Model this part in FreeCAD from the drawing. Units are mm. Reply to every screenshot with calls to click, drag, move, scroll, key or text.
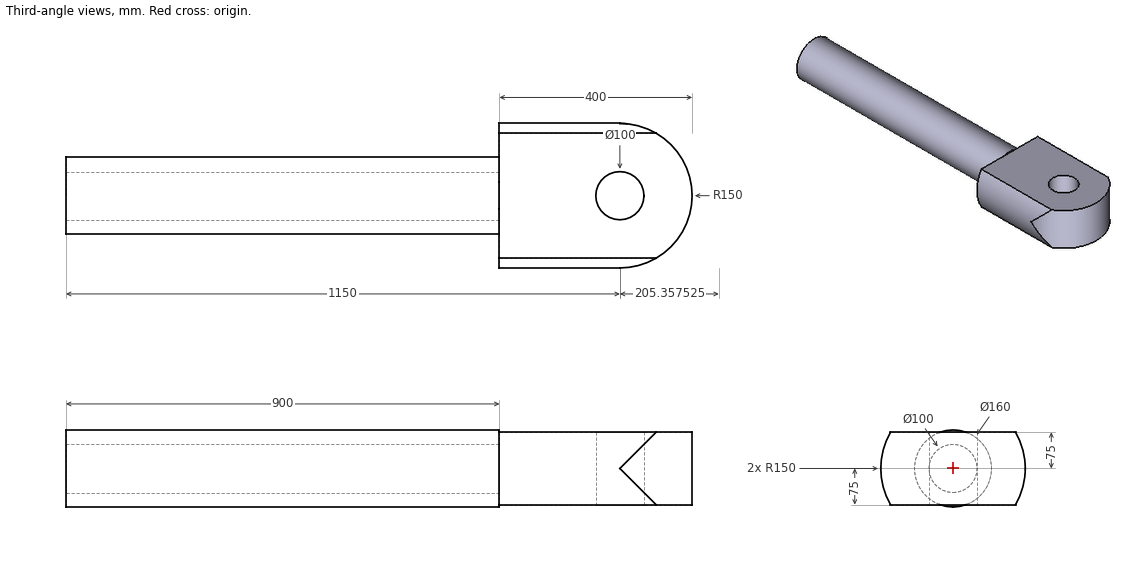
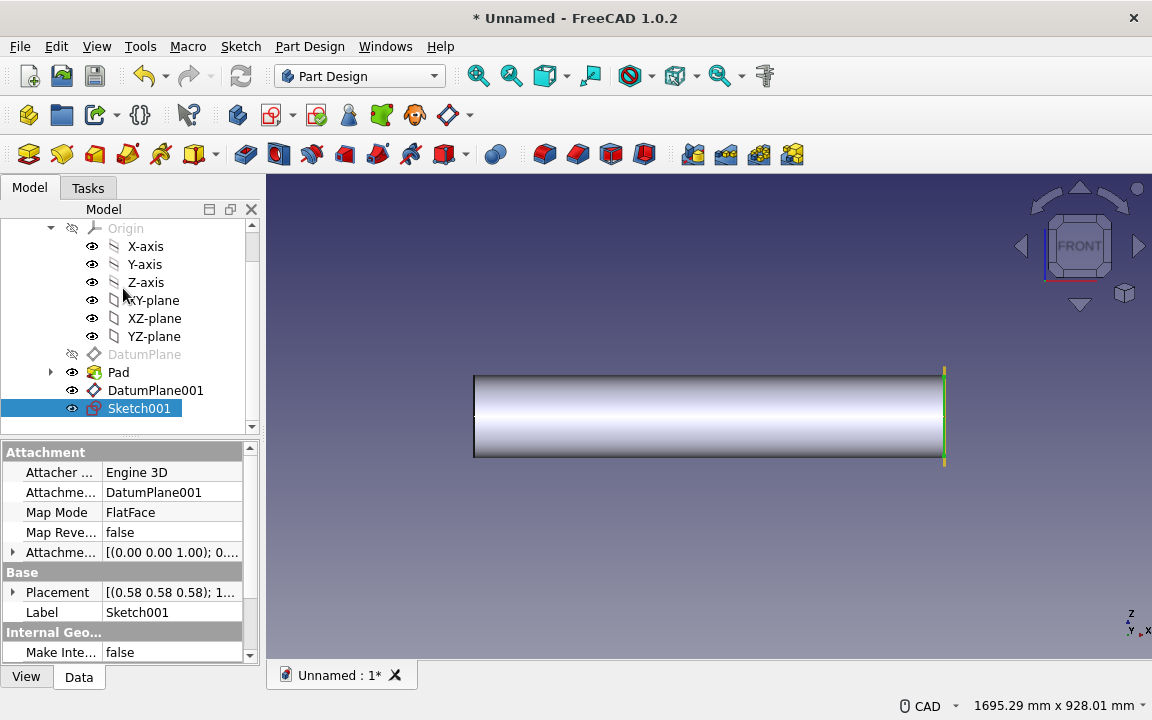
click(29, 154)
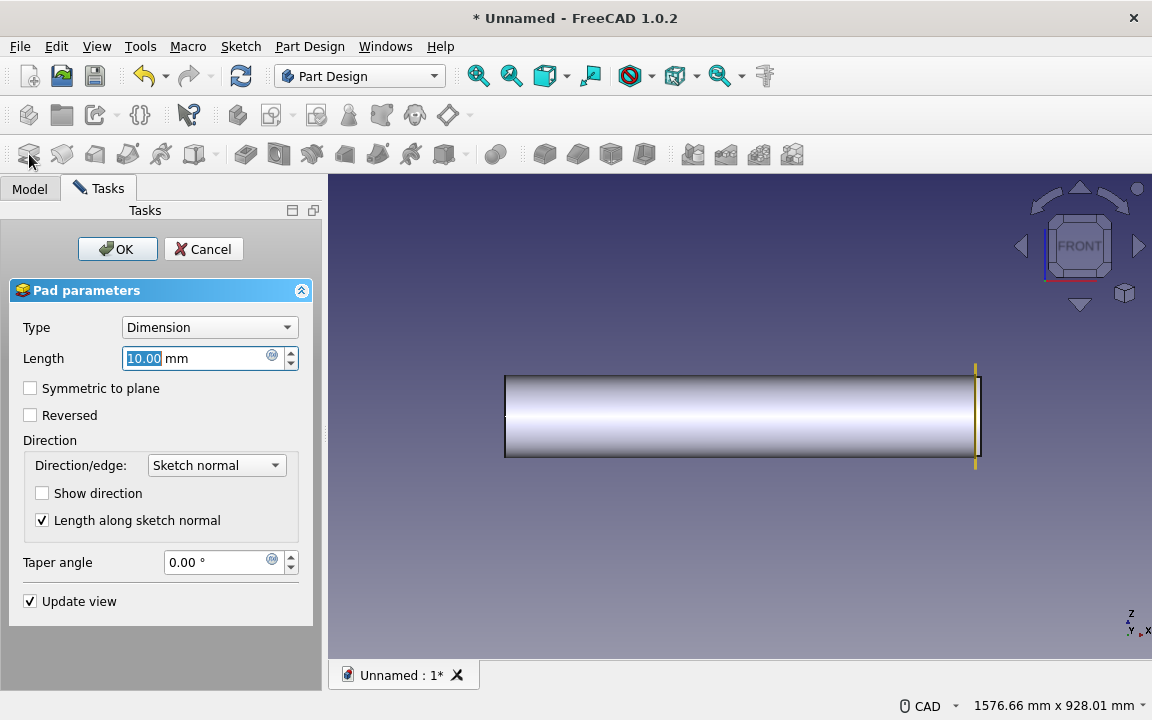
text(400)
key(Tab)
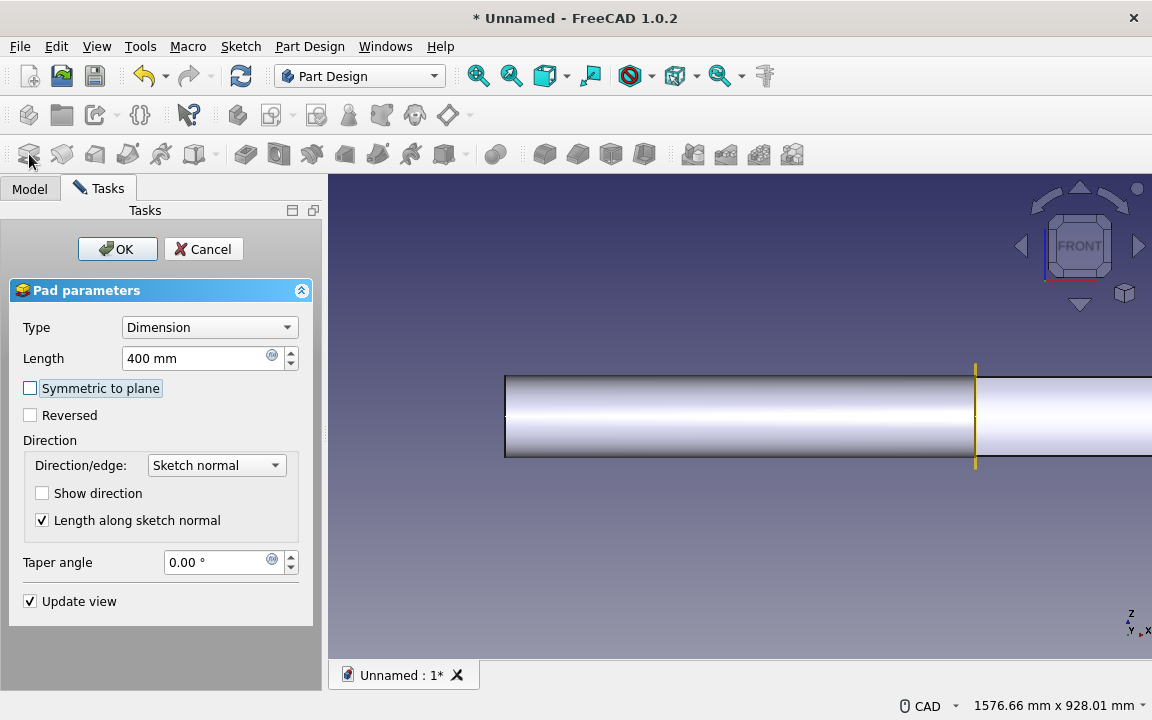
click(118, 249)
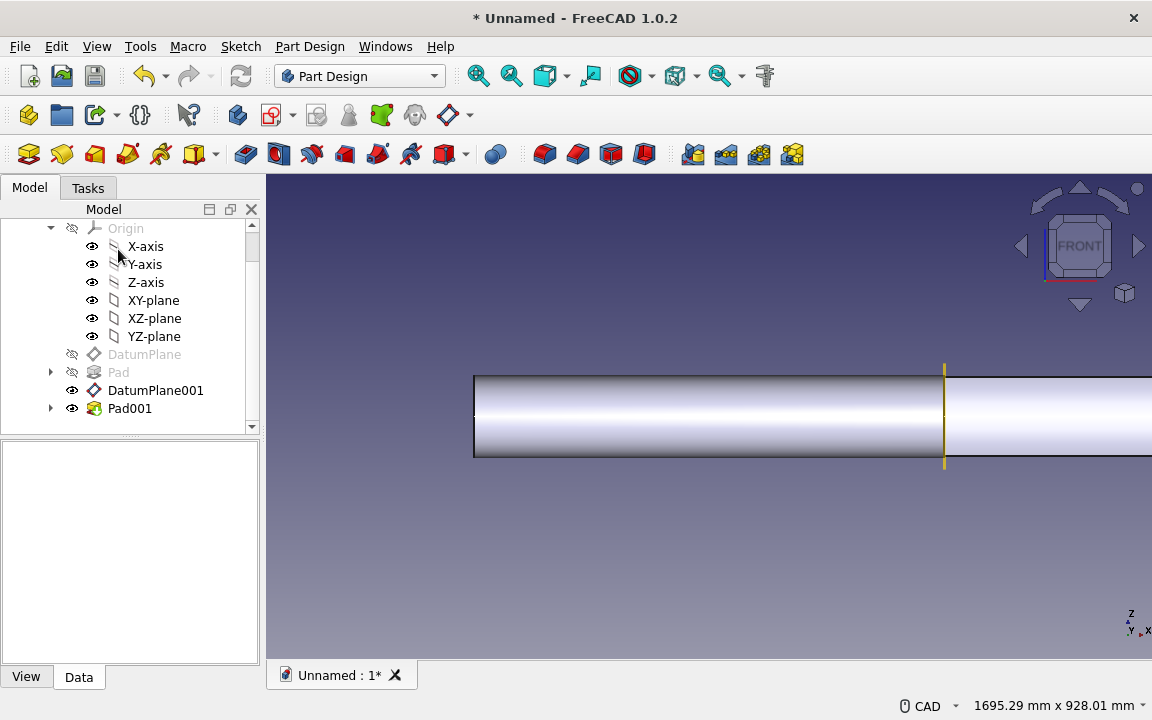
click(117, 390)
key(space)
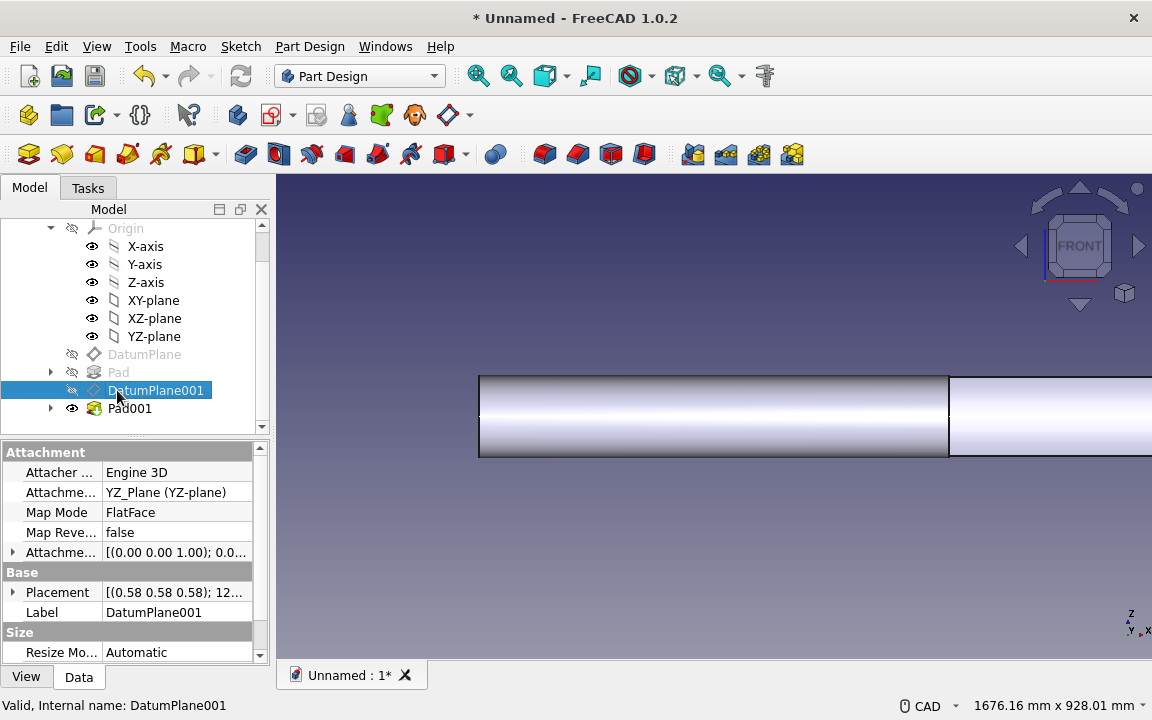
key(v)
key(f)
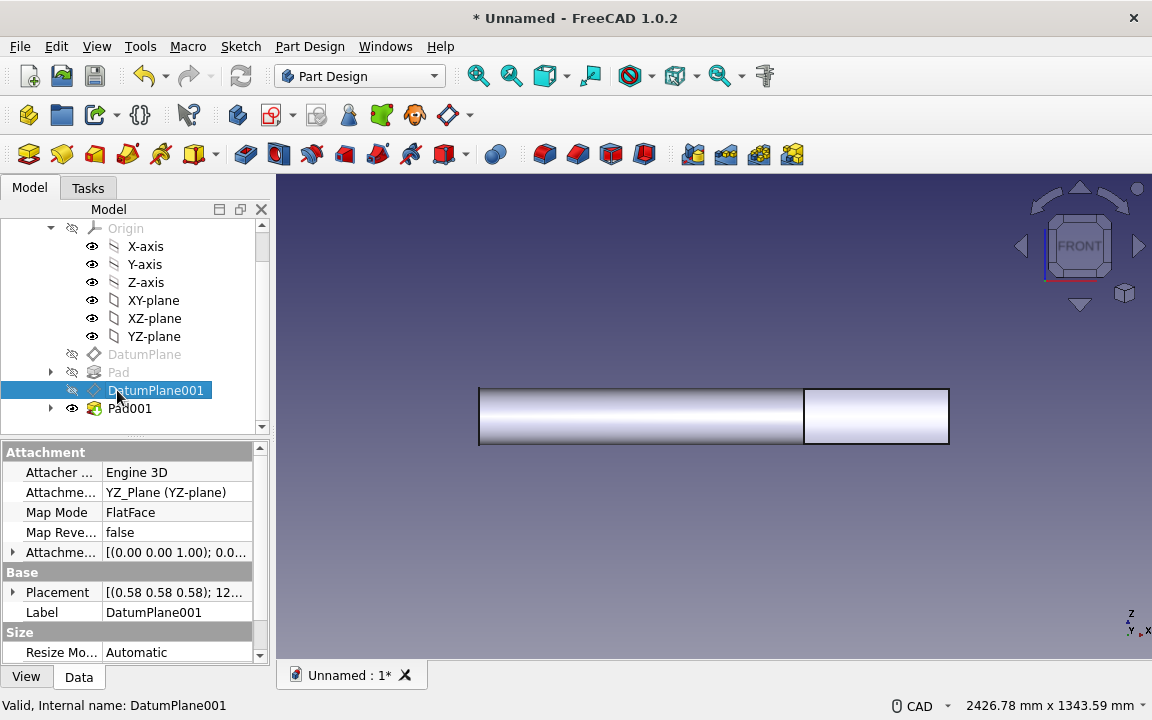
key(0)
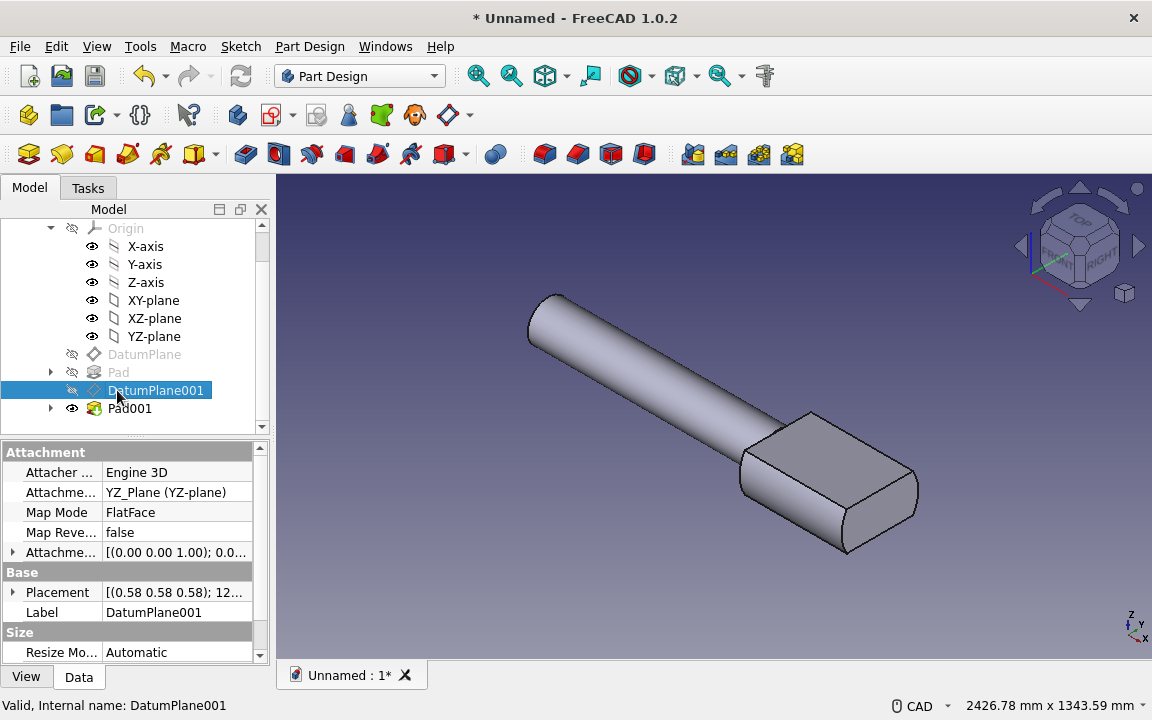
click(843, 468)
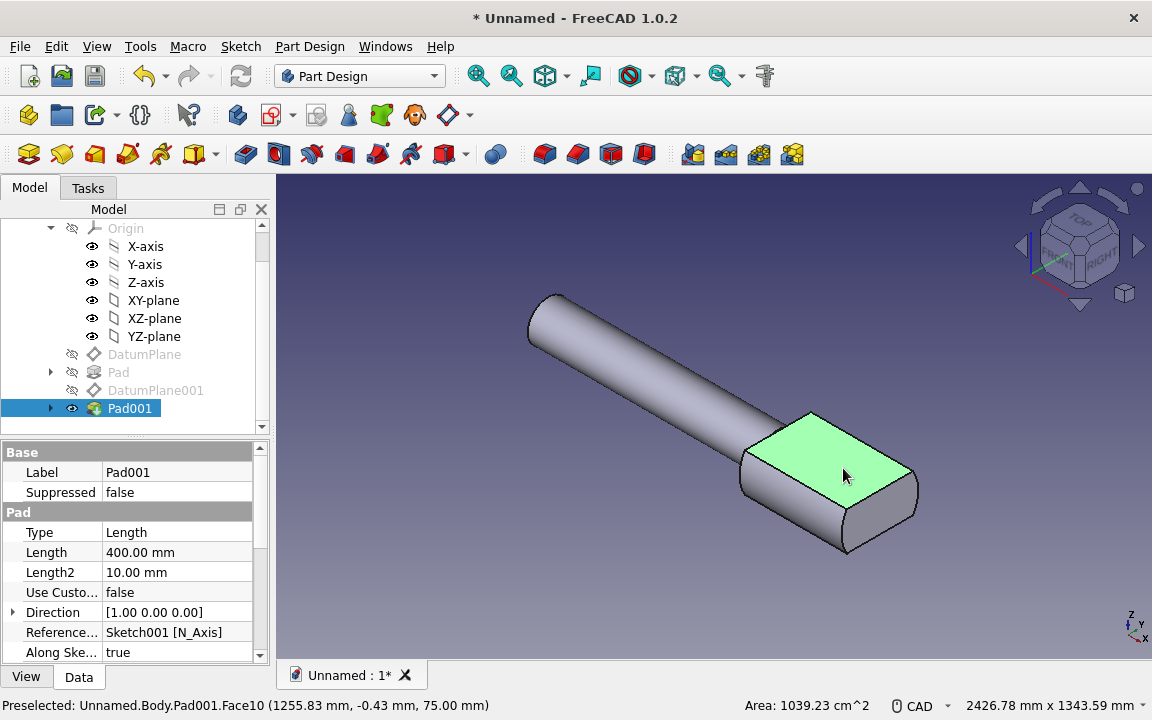
click(270, 116)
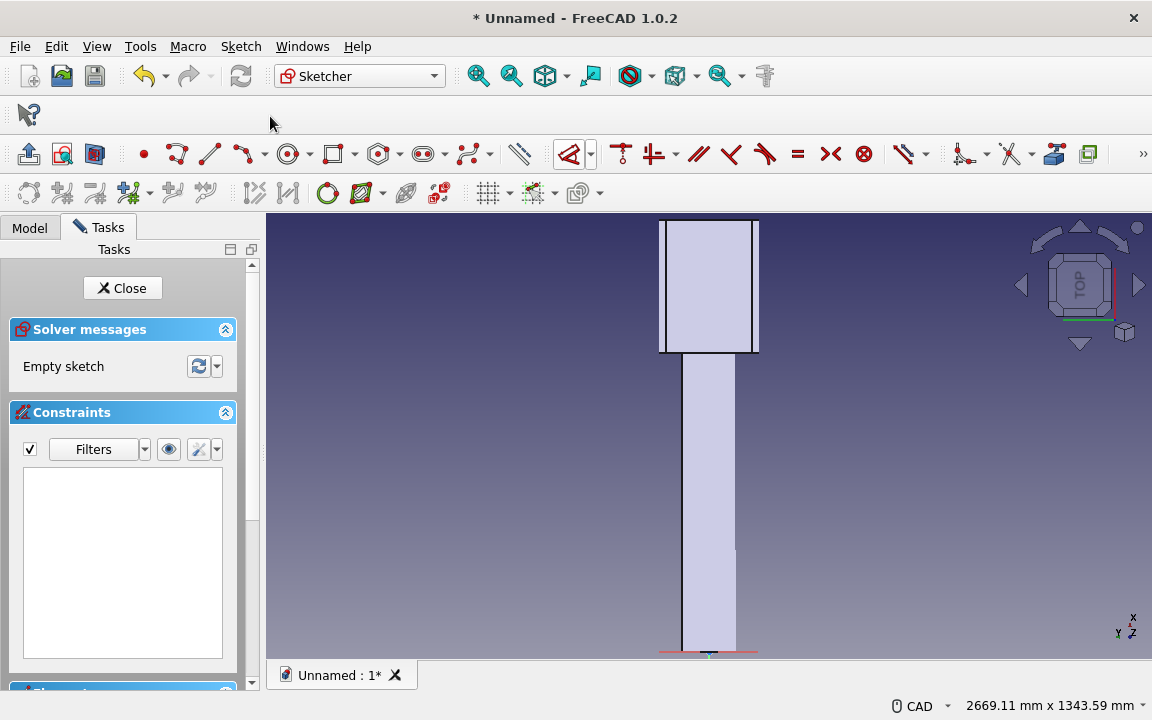
key(q)
key(s)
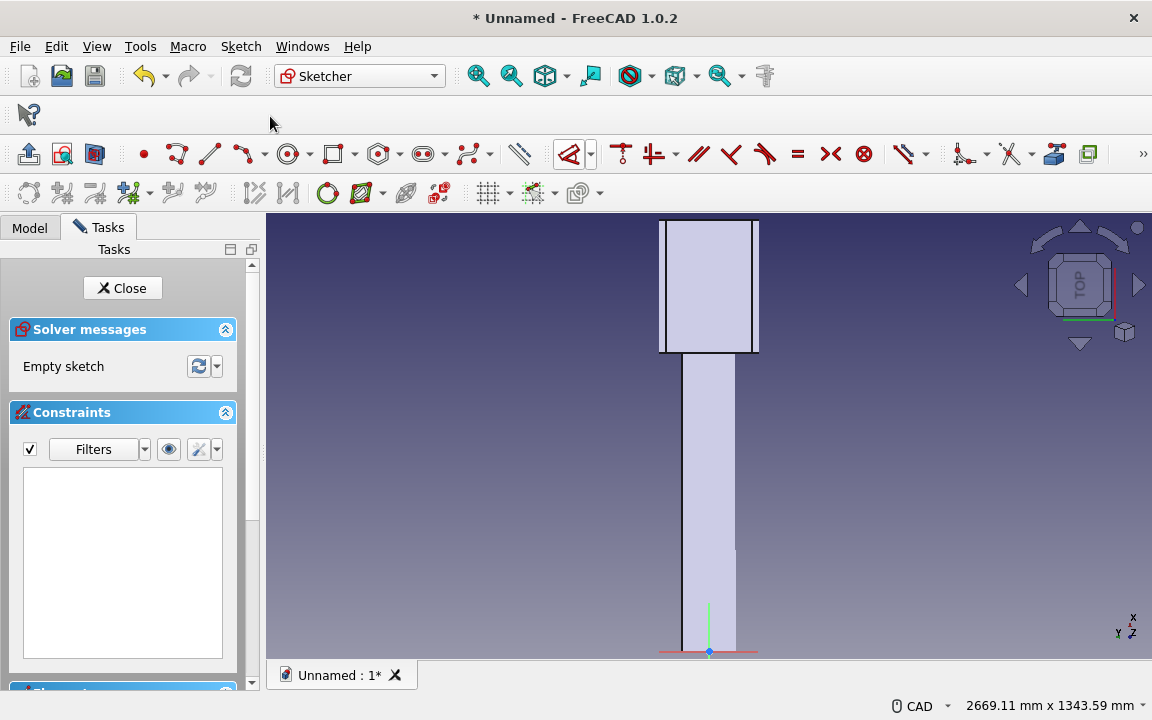
scroll(640, 436, down, 5)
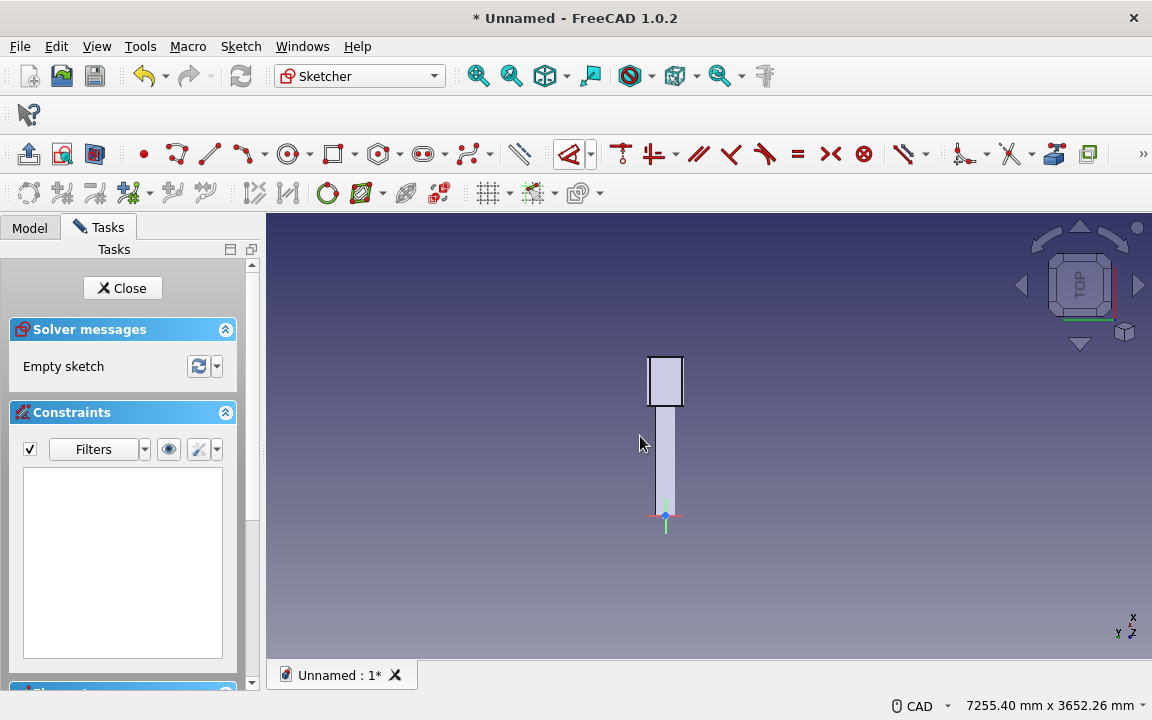
scroll(668, 355, up, 12)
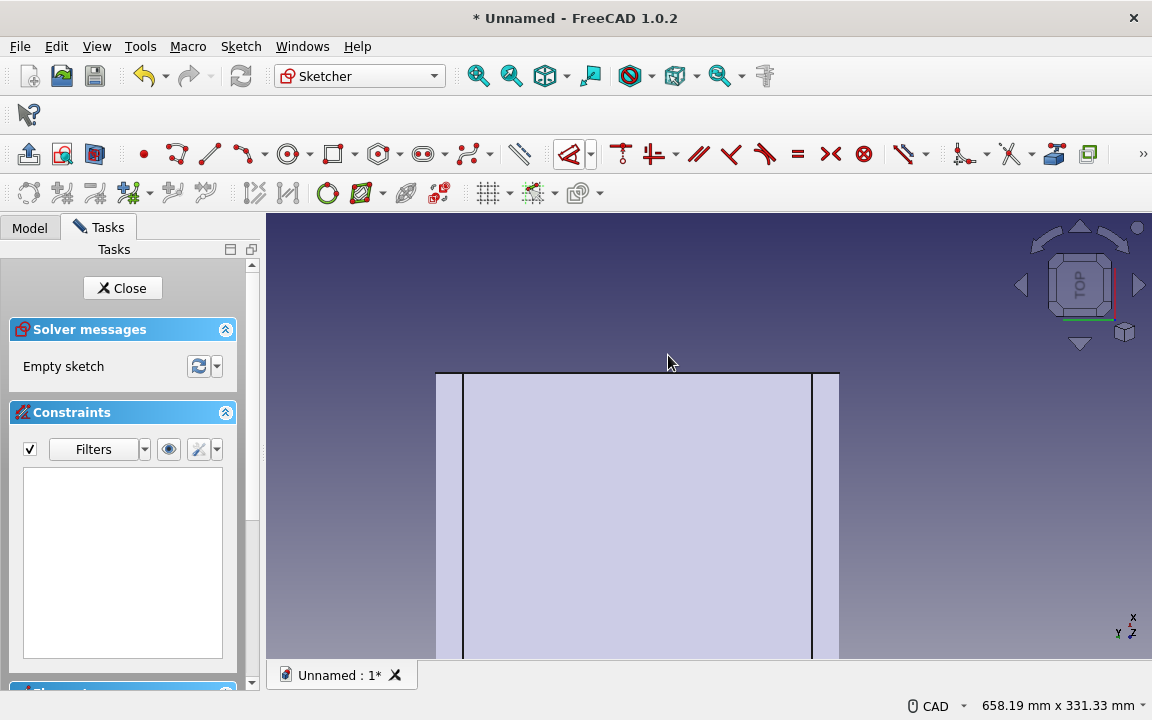
click(177, 154)